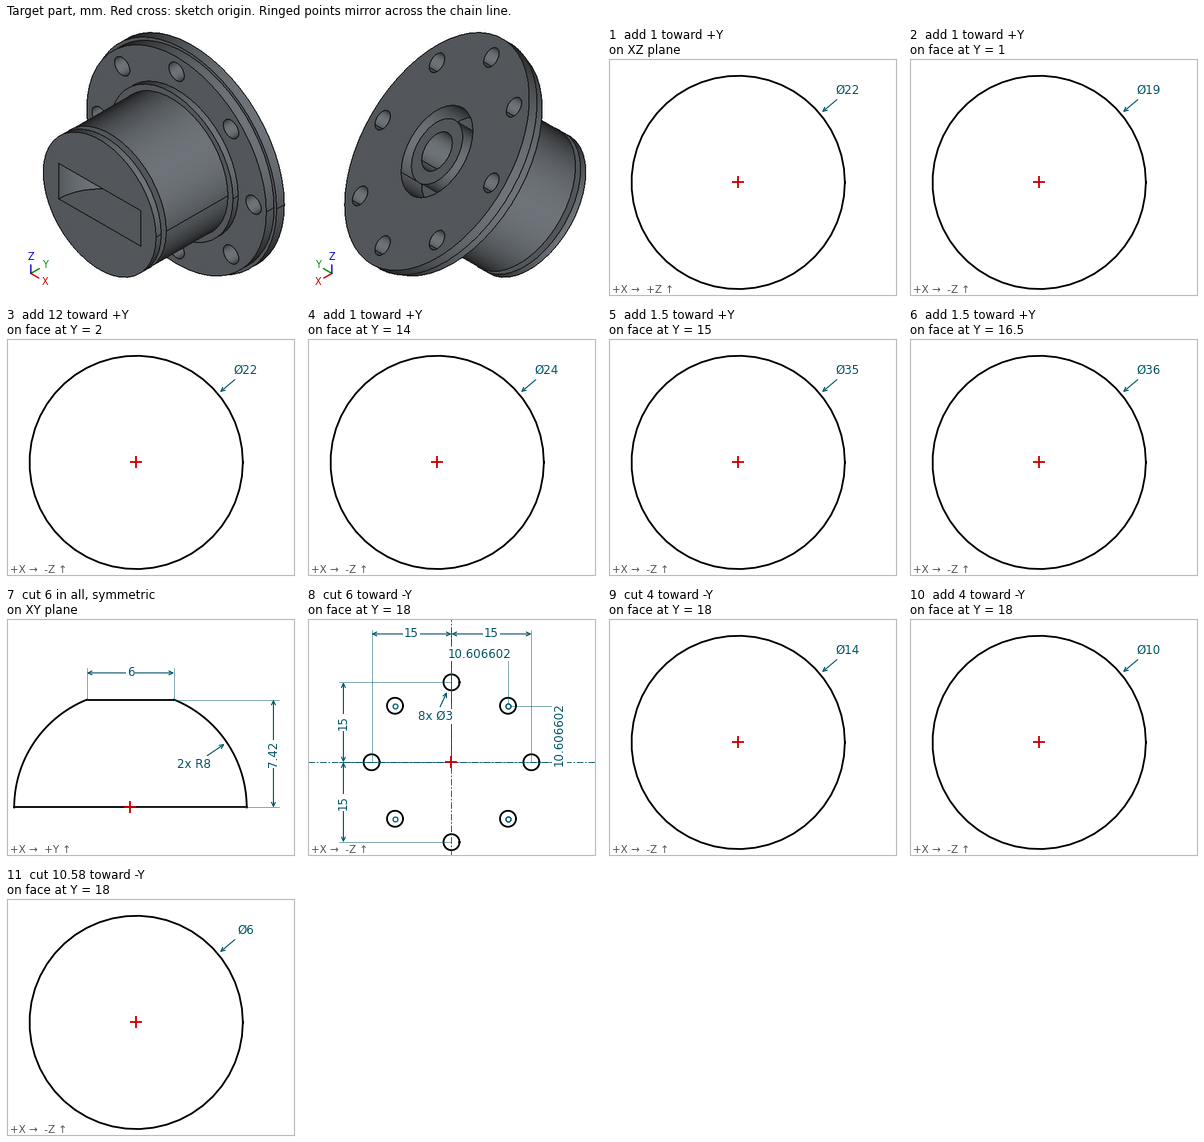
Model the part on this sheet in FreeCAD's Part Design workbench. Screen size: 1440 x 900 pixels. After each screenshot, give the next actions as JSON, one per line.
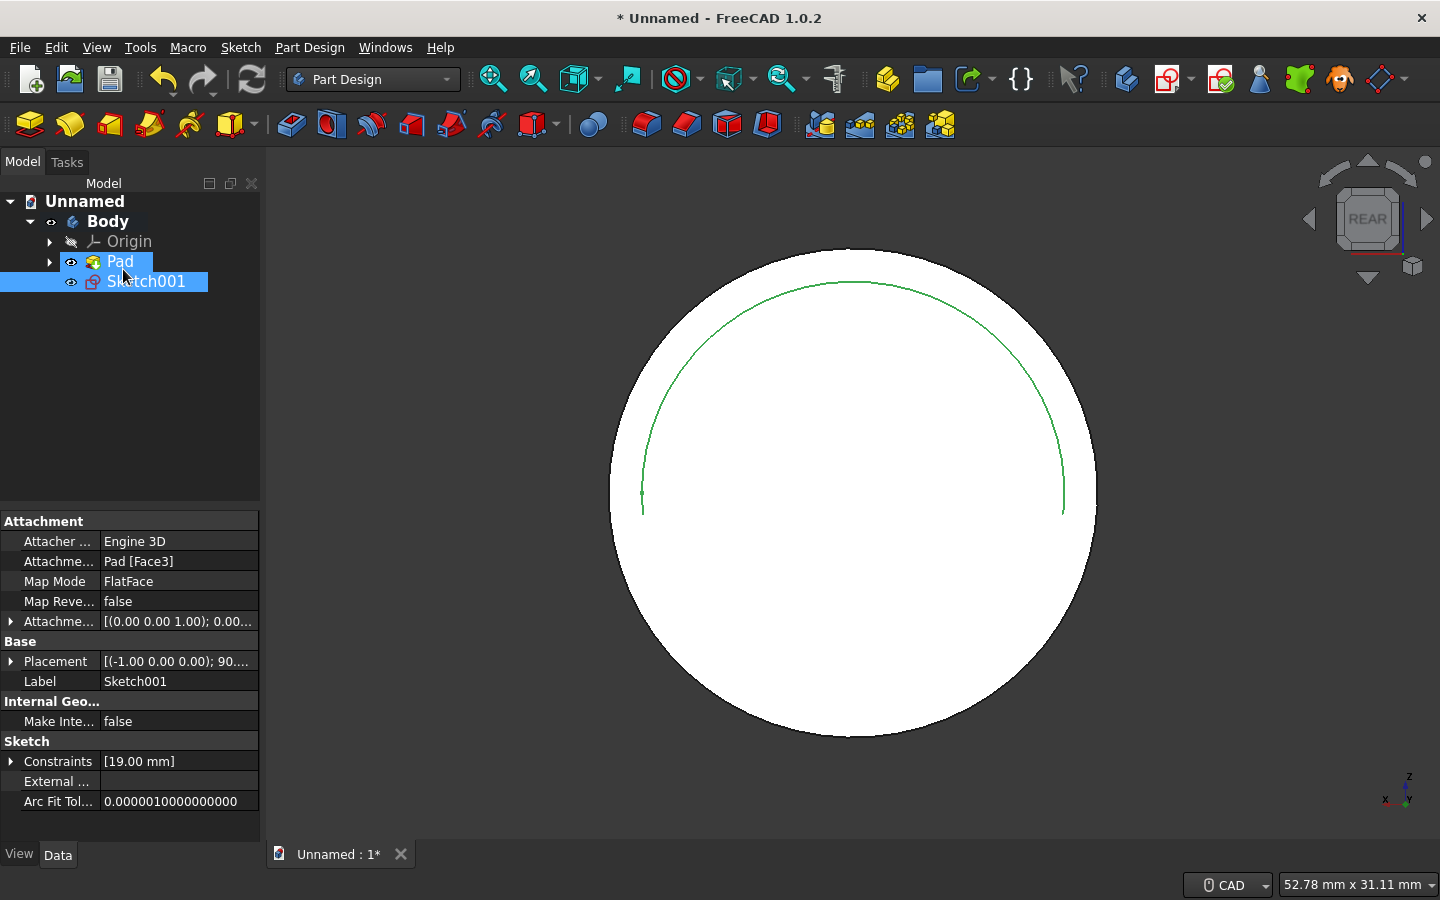
{"action": "left_click", "coordinate": [30, 124]}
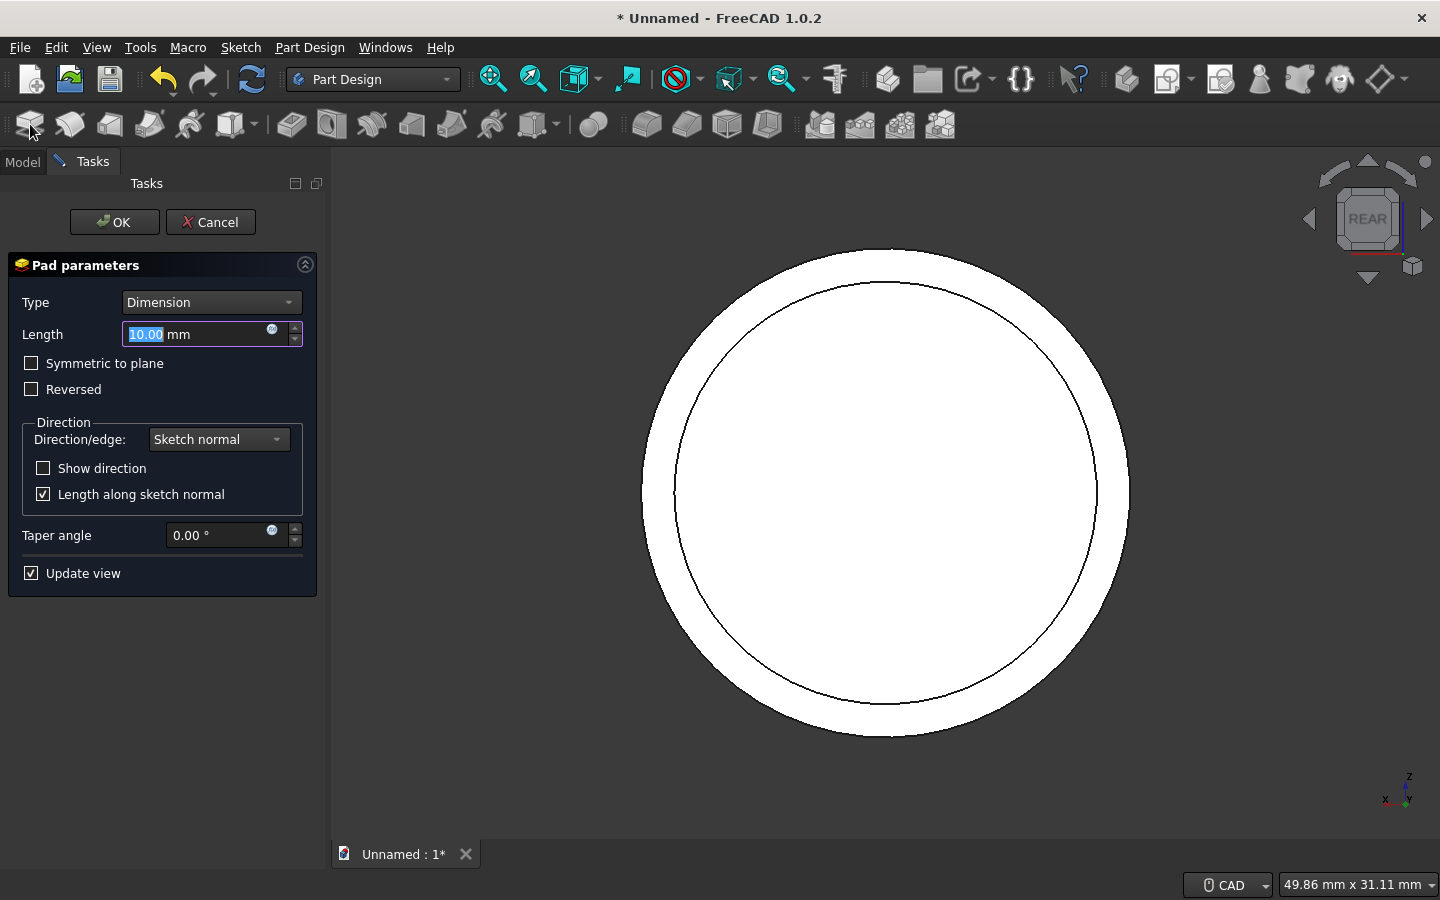
{"action": "type", "text": "1"}
{"action": "key", "text": "Tab"}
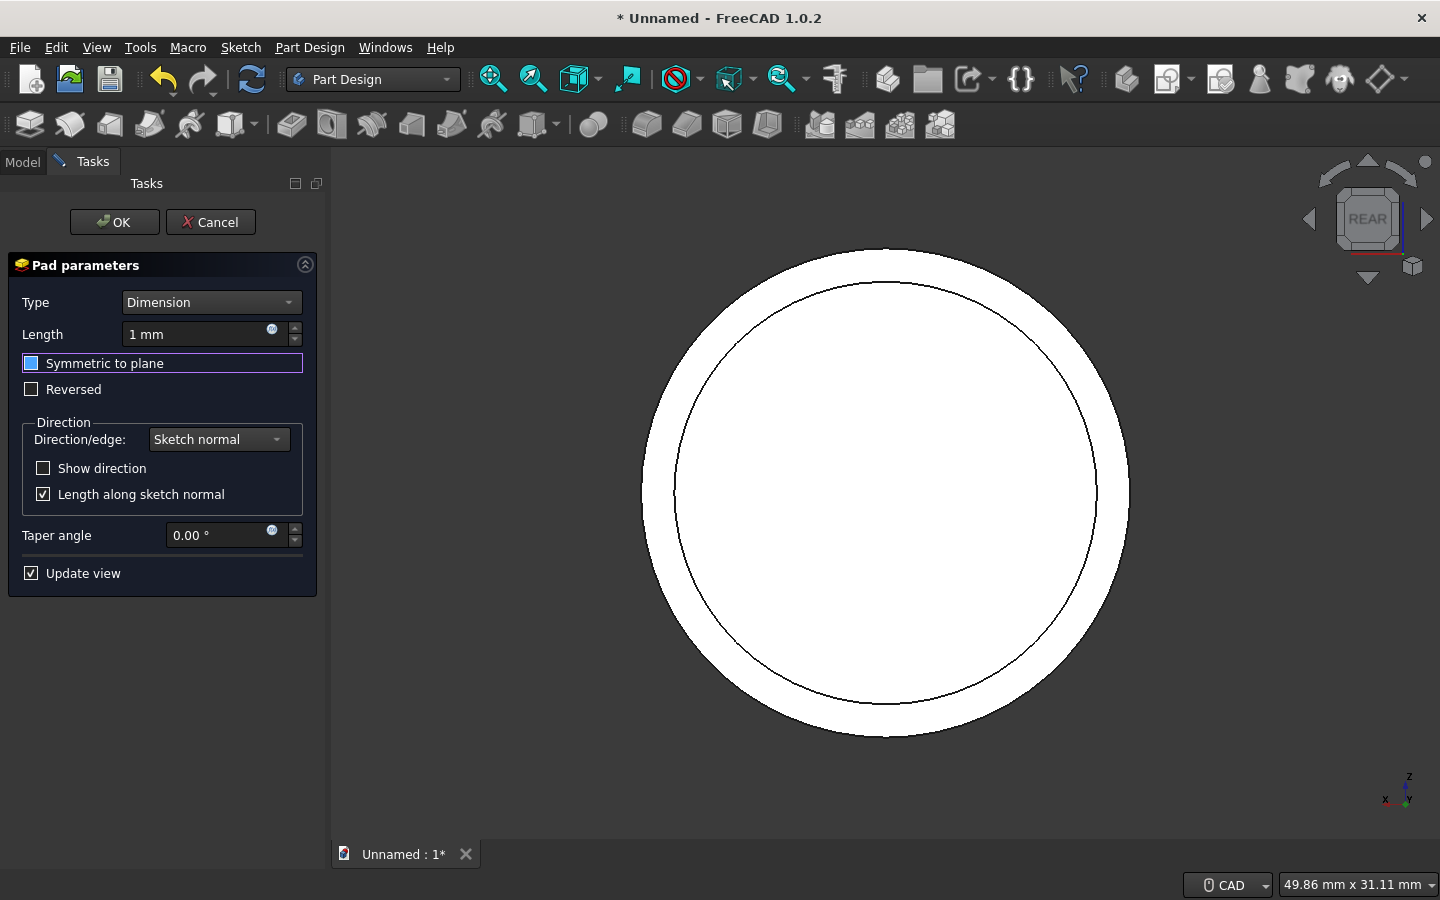
{"action": "left_click", "coordinate": [115, 222]}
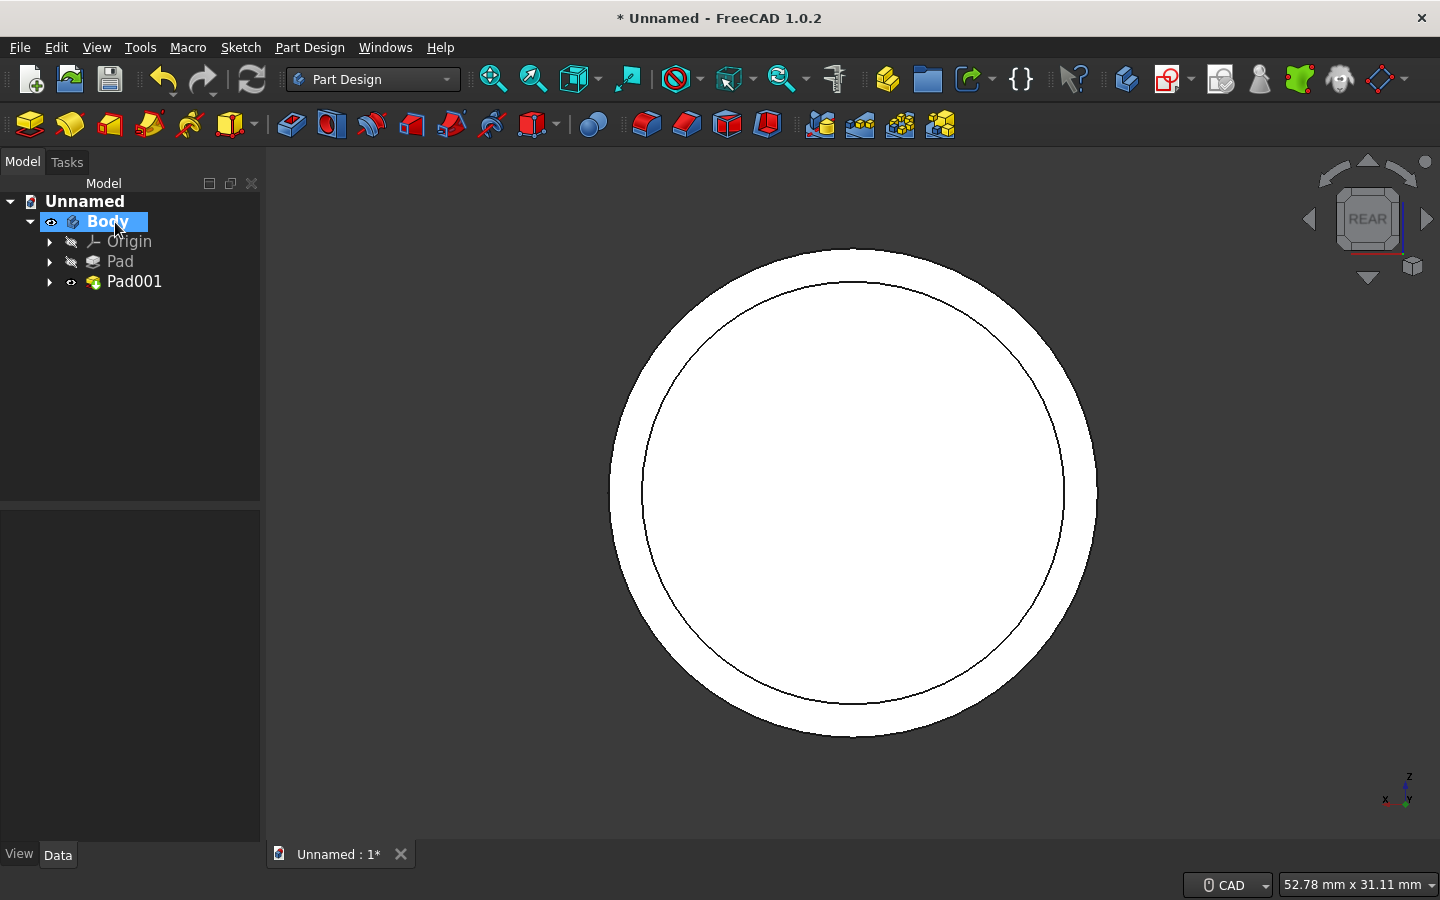
{"action": "left_click", "coordinate": [853, 492]}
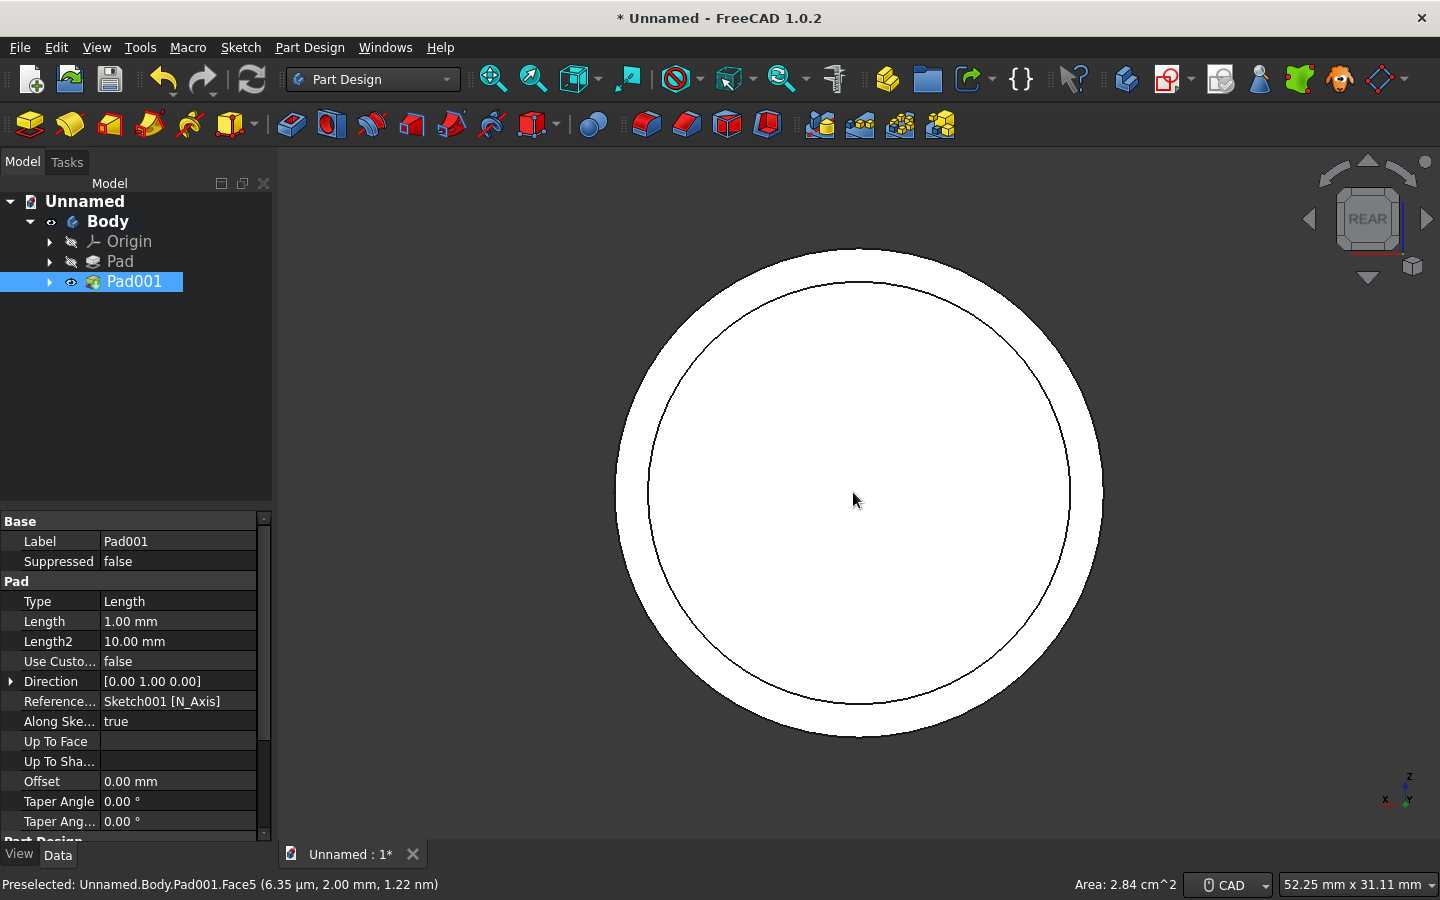
{"action": "left_click", "coordinate": [1168, 80]}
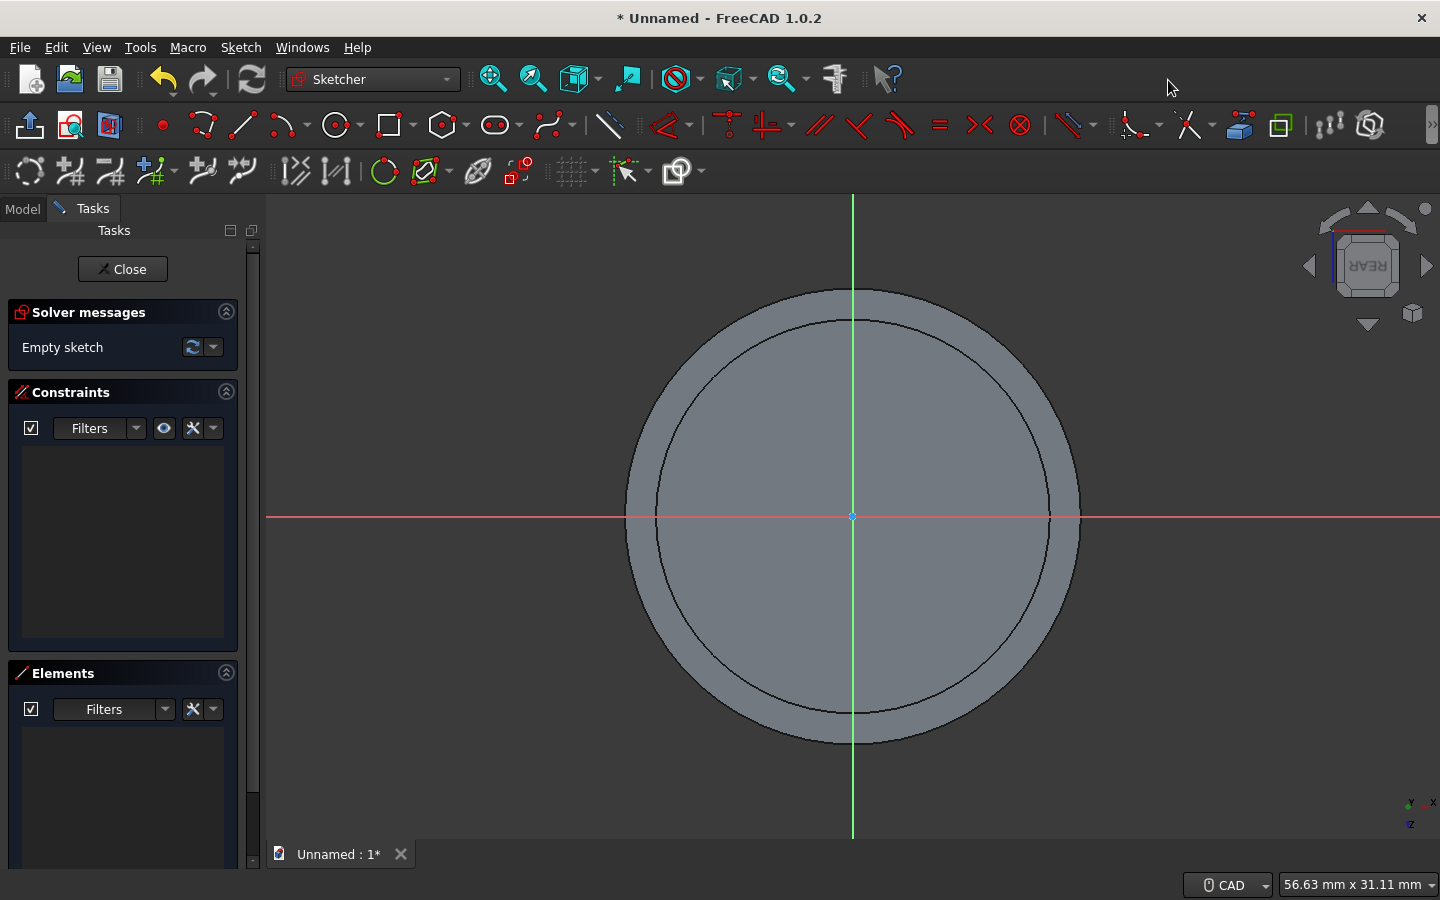
{"action": "left_click", "coordinate": [336, 126]}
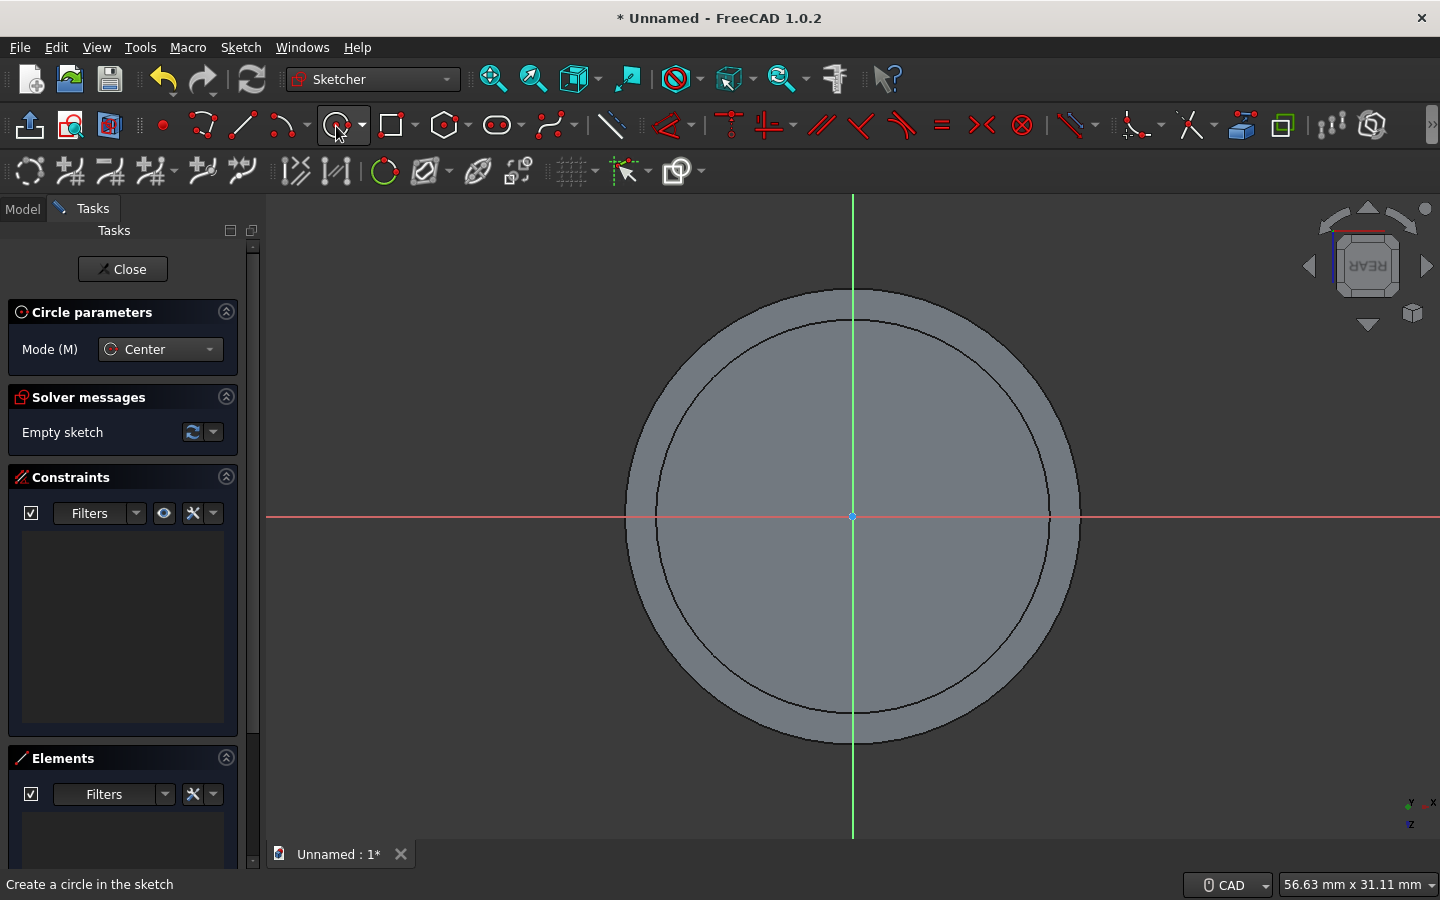
{"action": "left_click", "coordinate": [853, 516]}
{"action": "mouse_move", "coordinate": [1014, 355]}